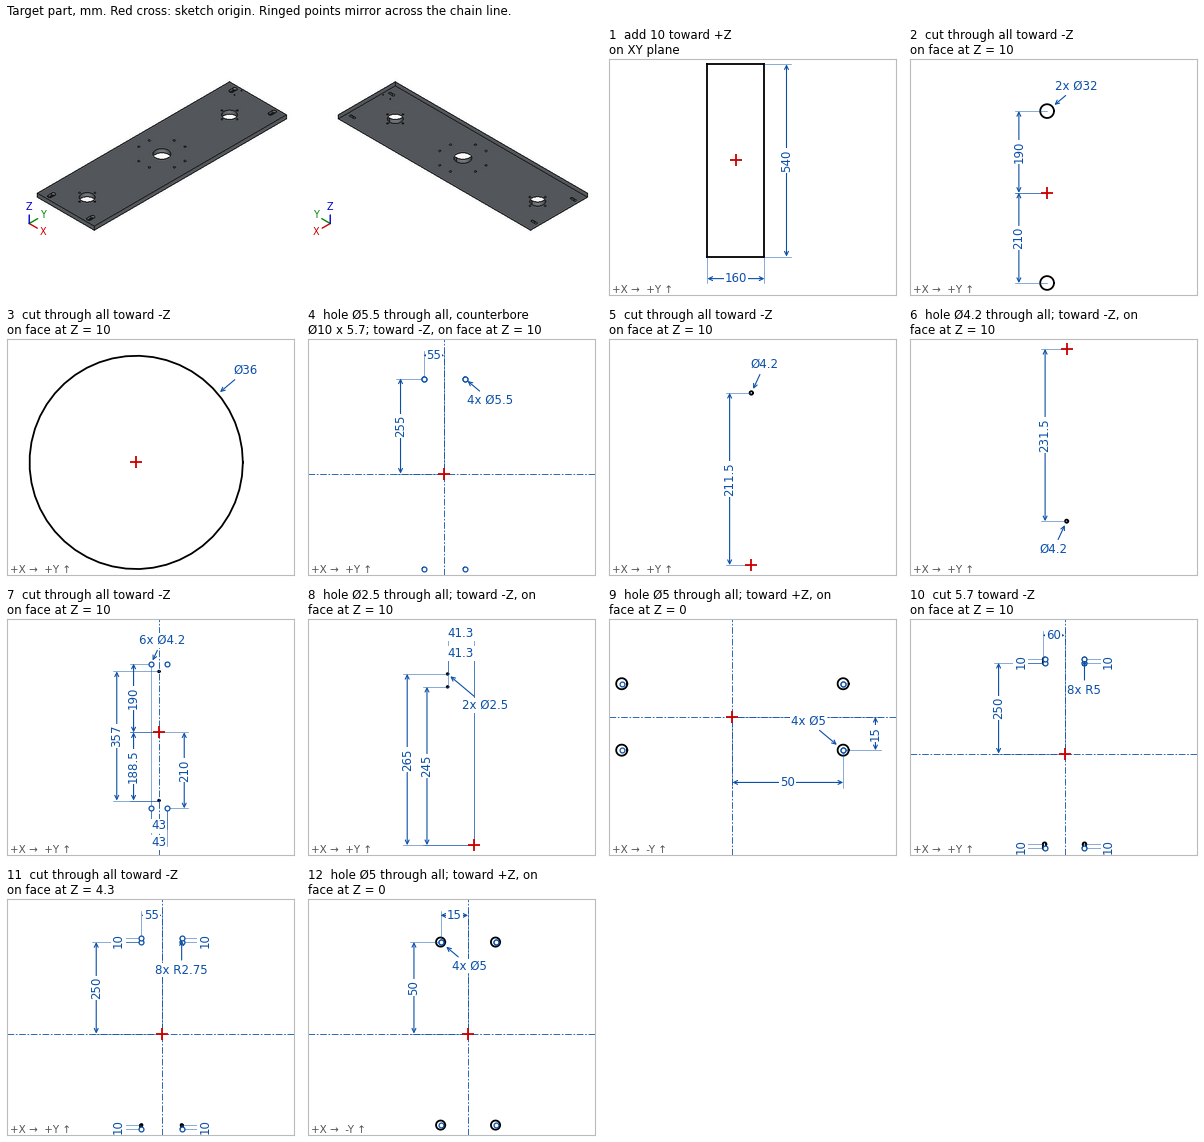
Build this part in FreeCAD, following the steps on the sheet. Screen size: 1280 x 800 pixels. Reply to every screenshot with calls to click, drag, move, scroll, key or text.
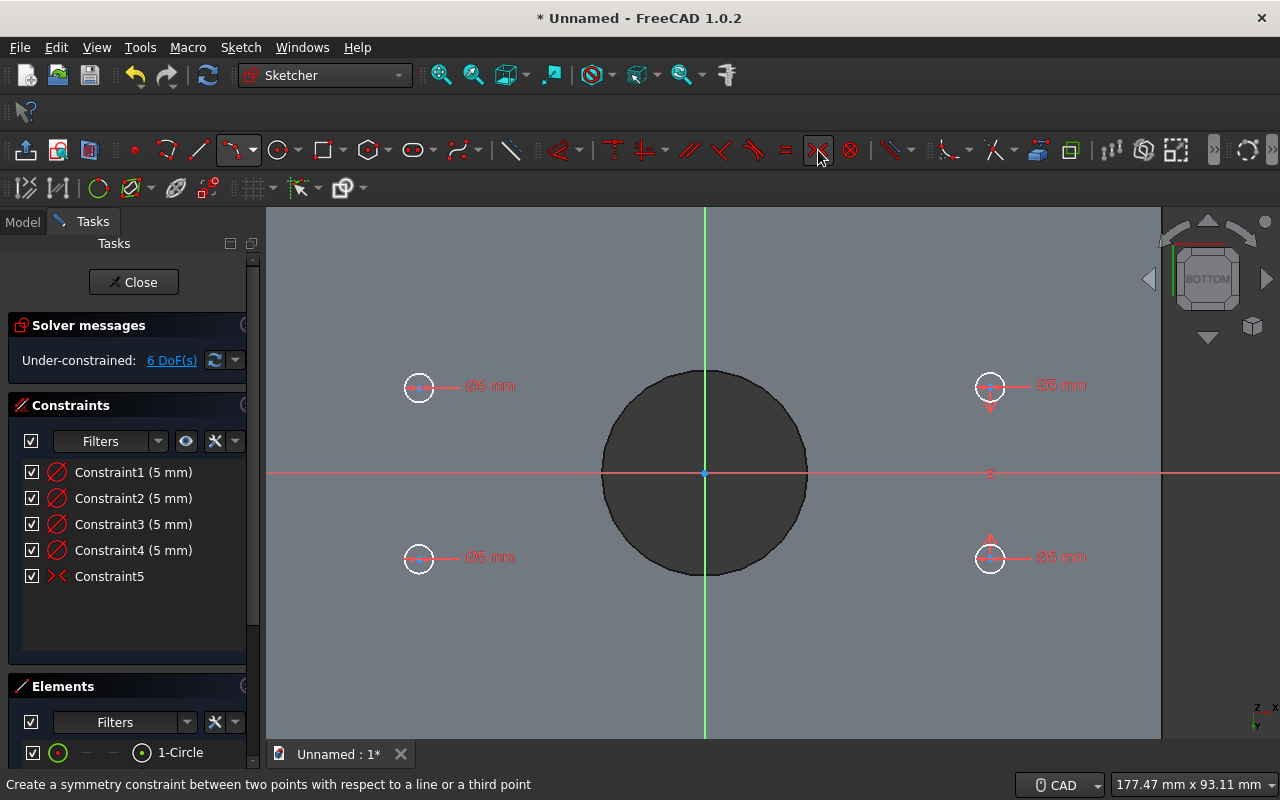
click(990, 559)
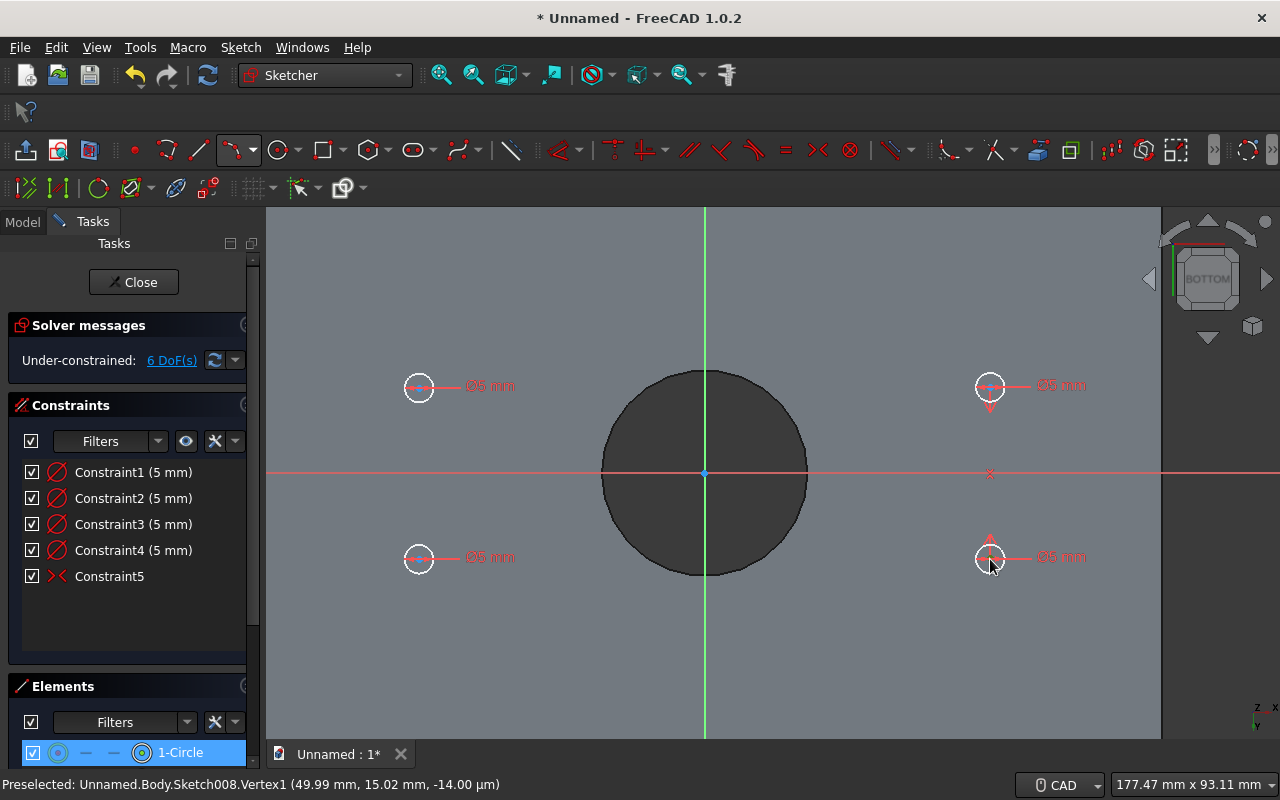
click(419, 559)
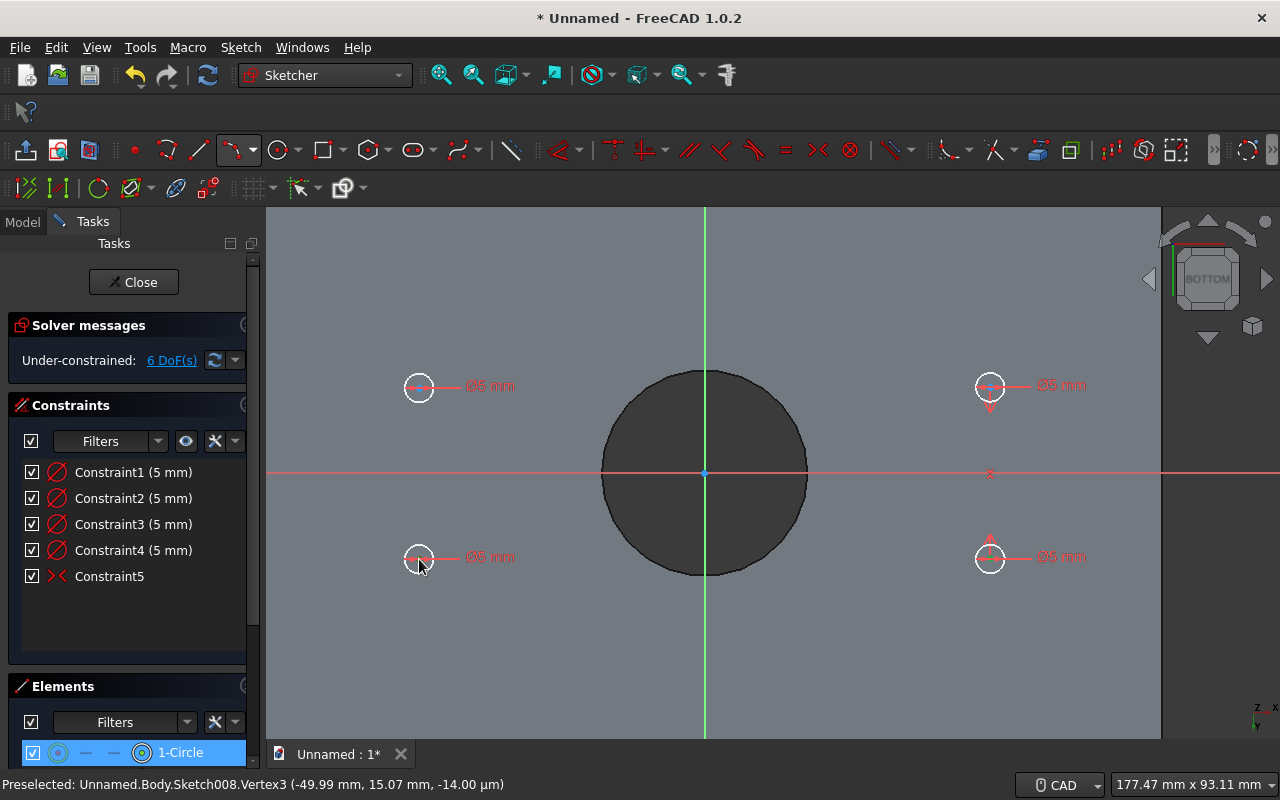
click(705, 677)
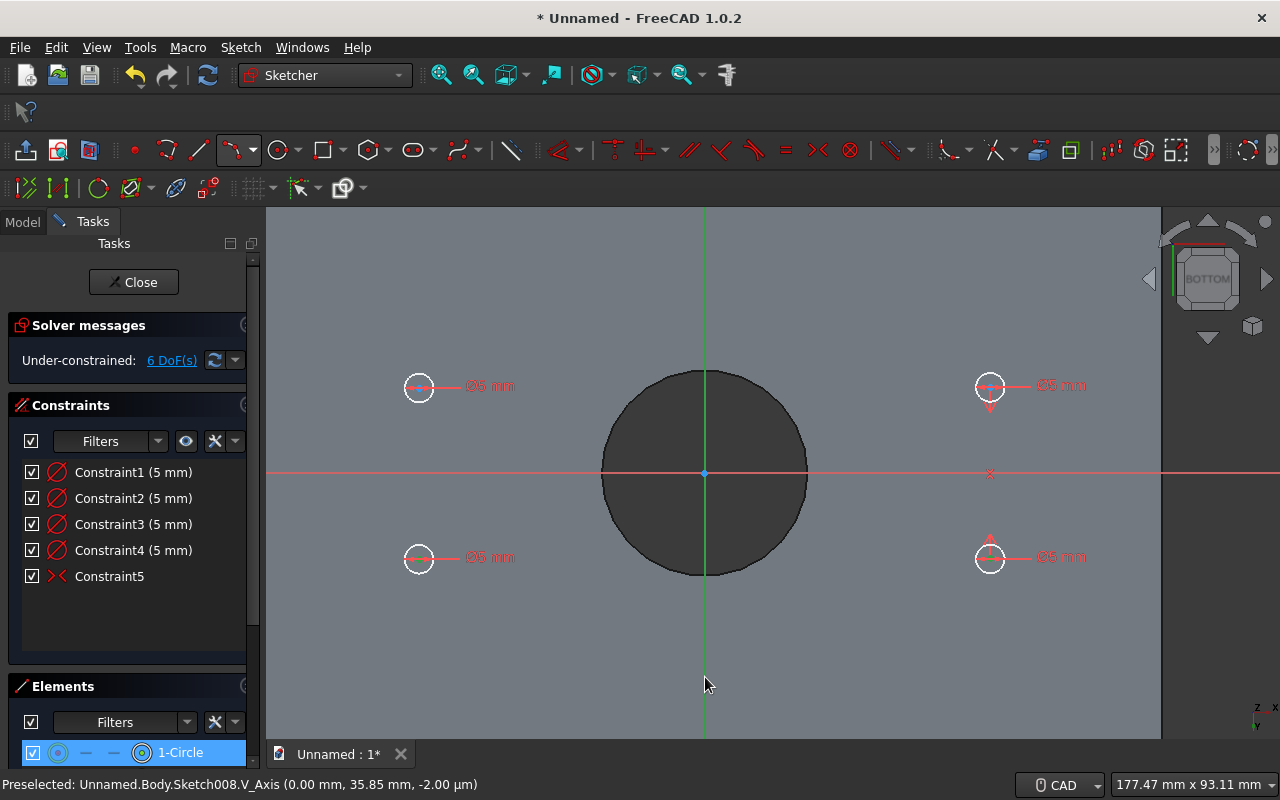
key(s)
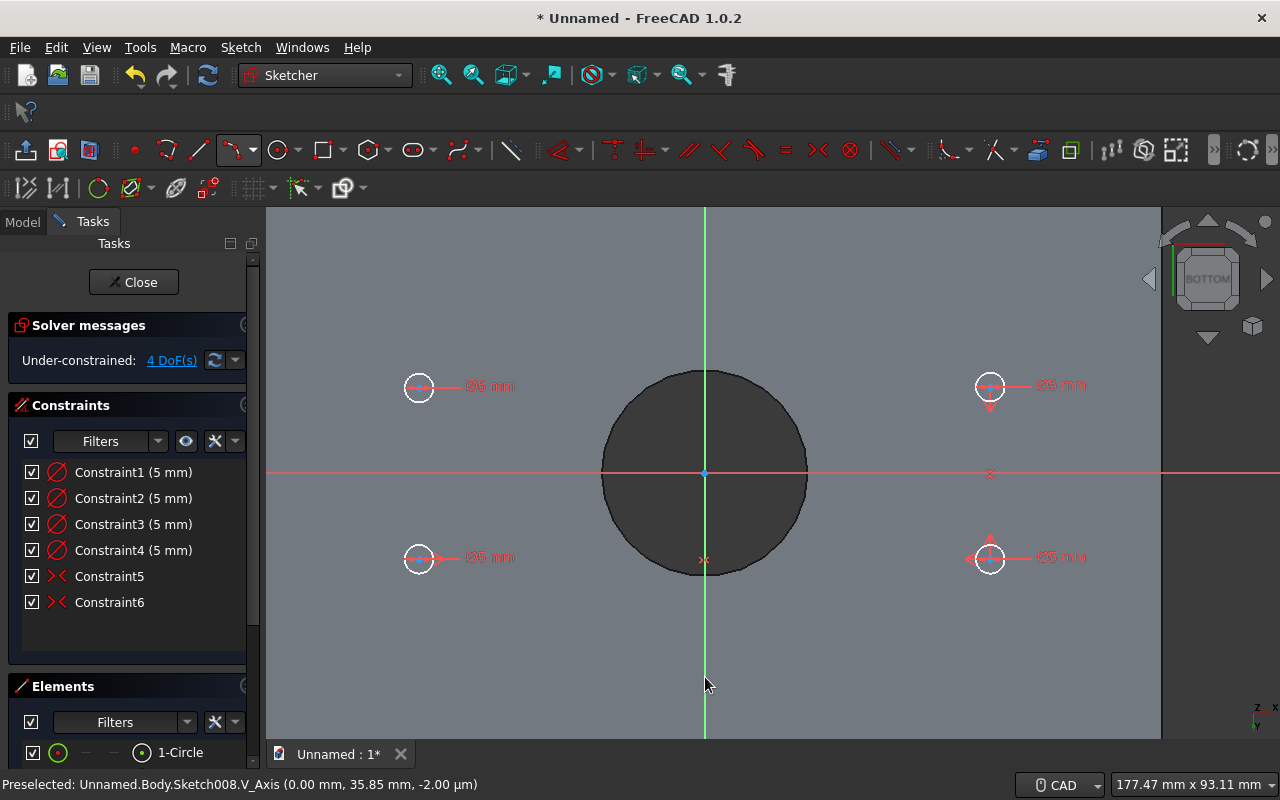
click(990, 387)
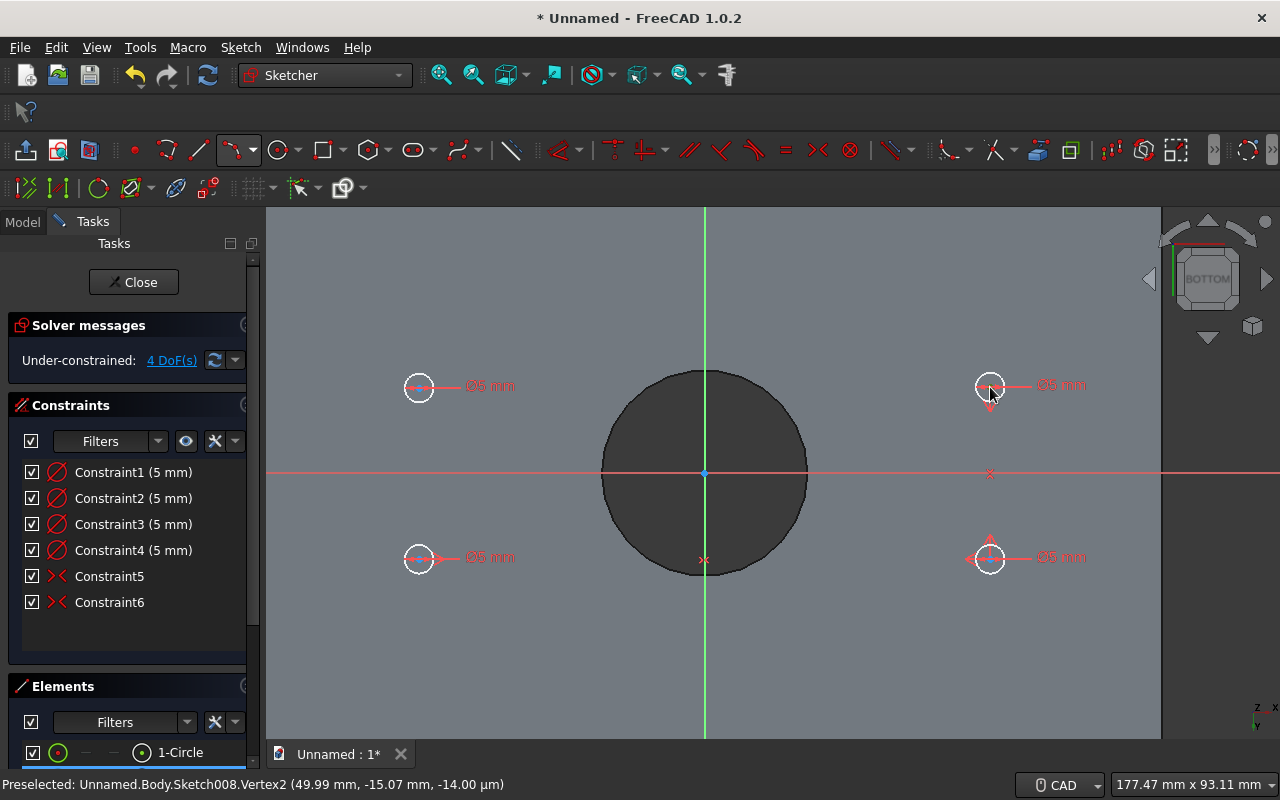
click(419, 388)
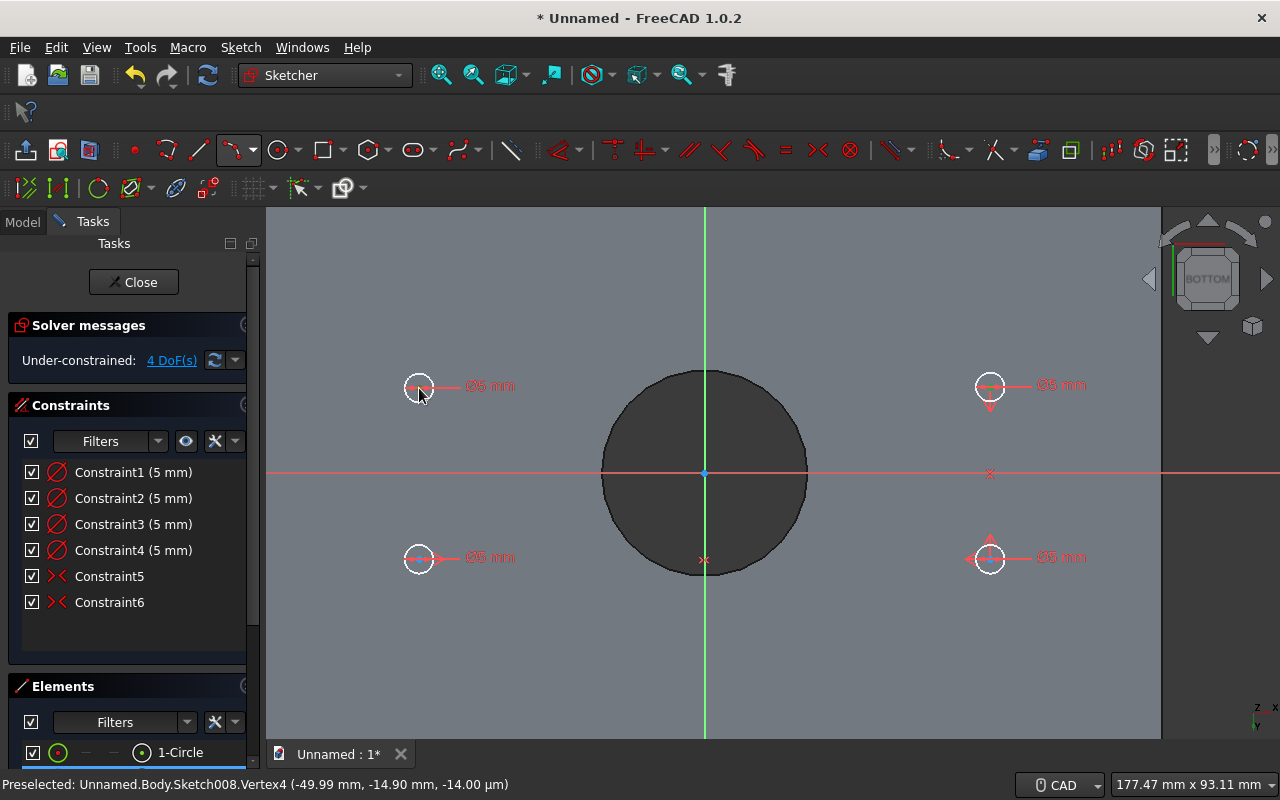
click(705, 677)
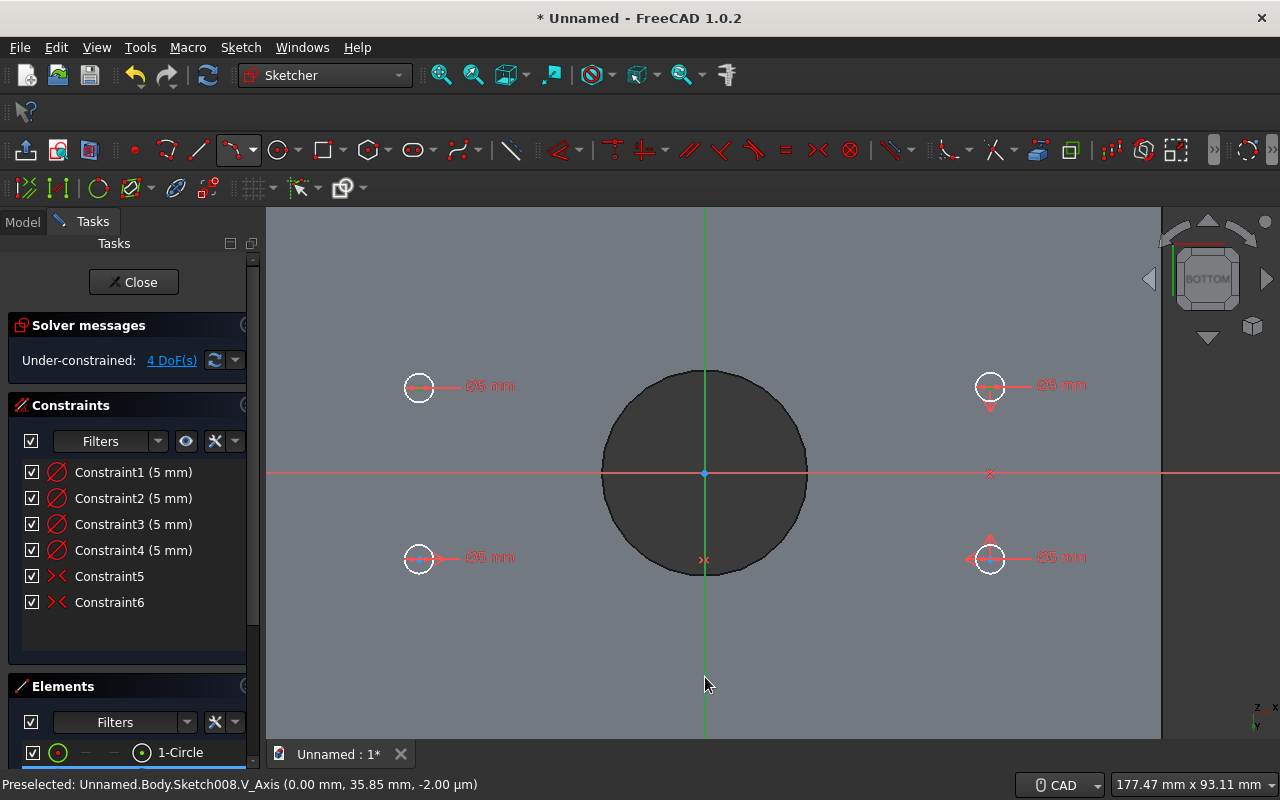
key(s)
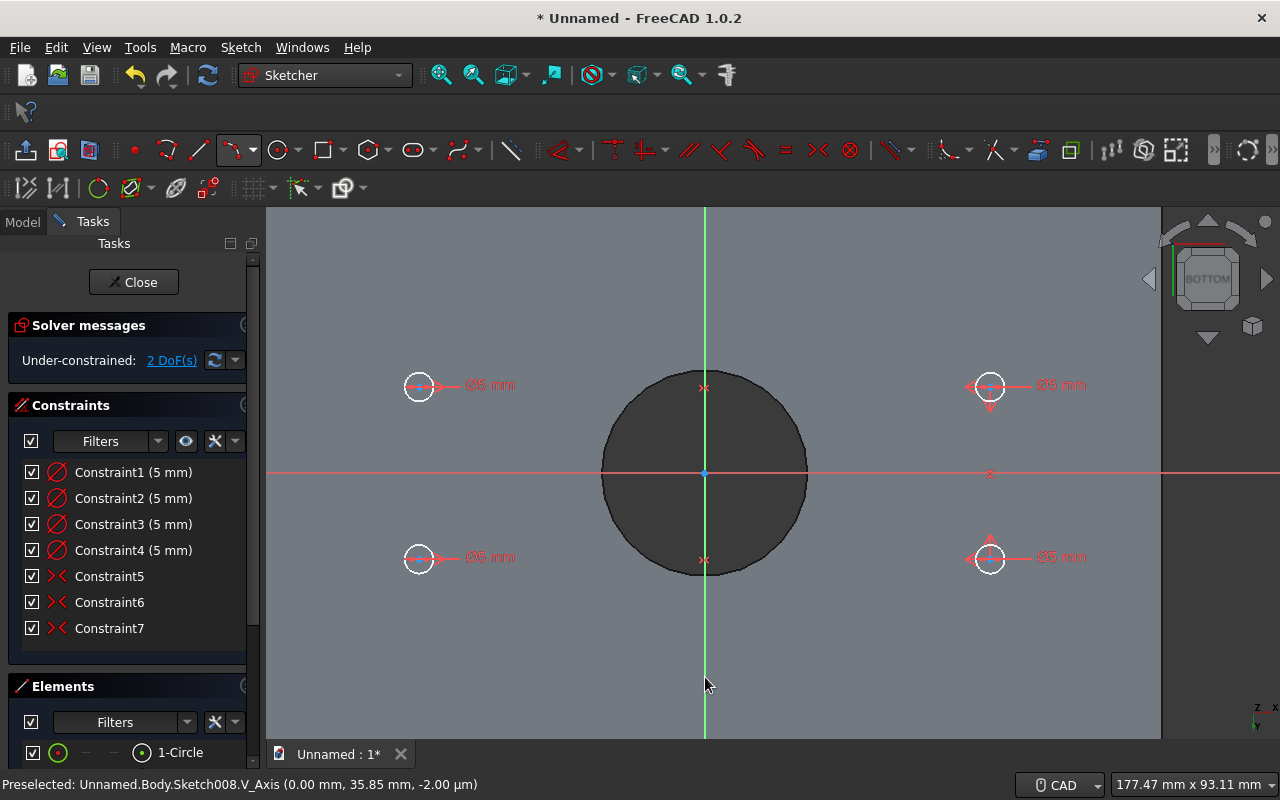
key(d)